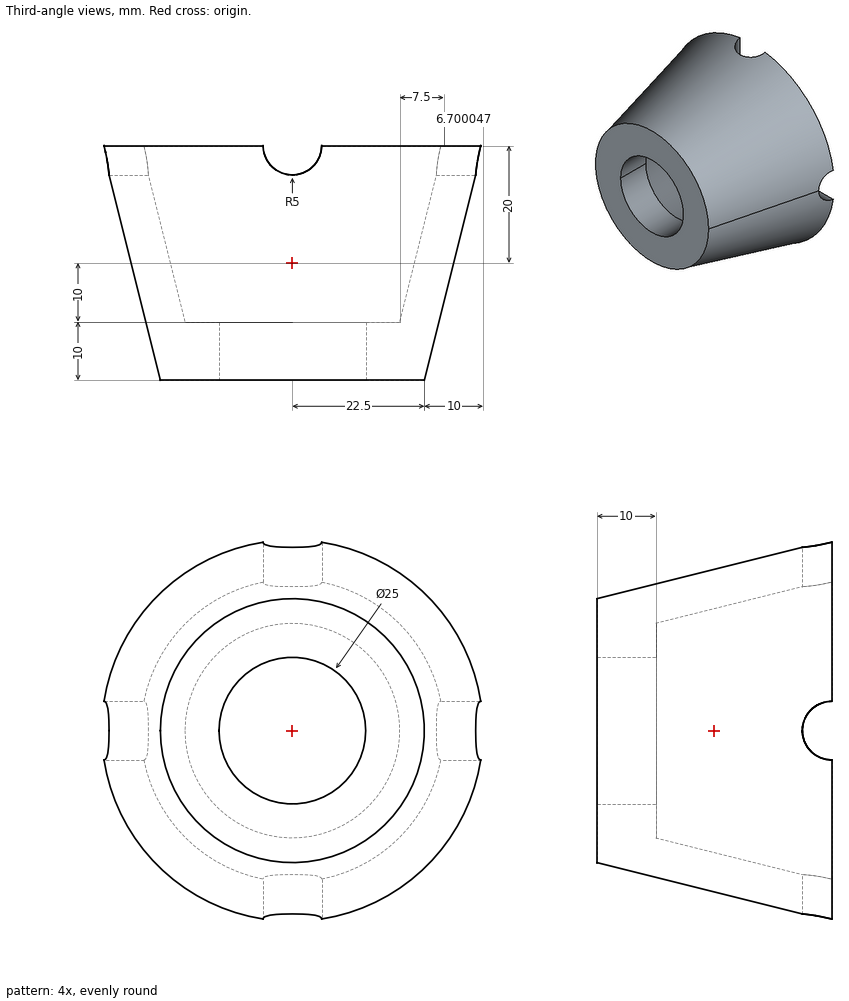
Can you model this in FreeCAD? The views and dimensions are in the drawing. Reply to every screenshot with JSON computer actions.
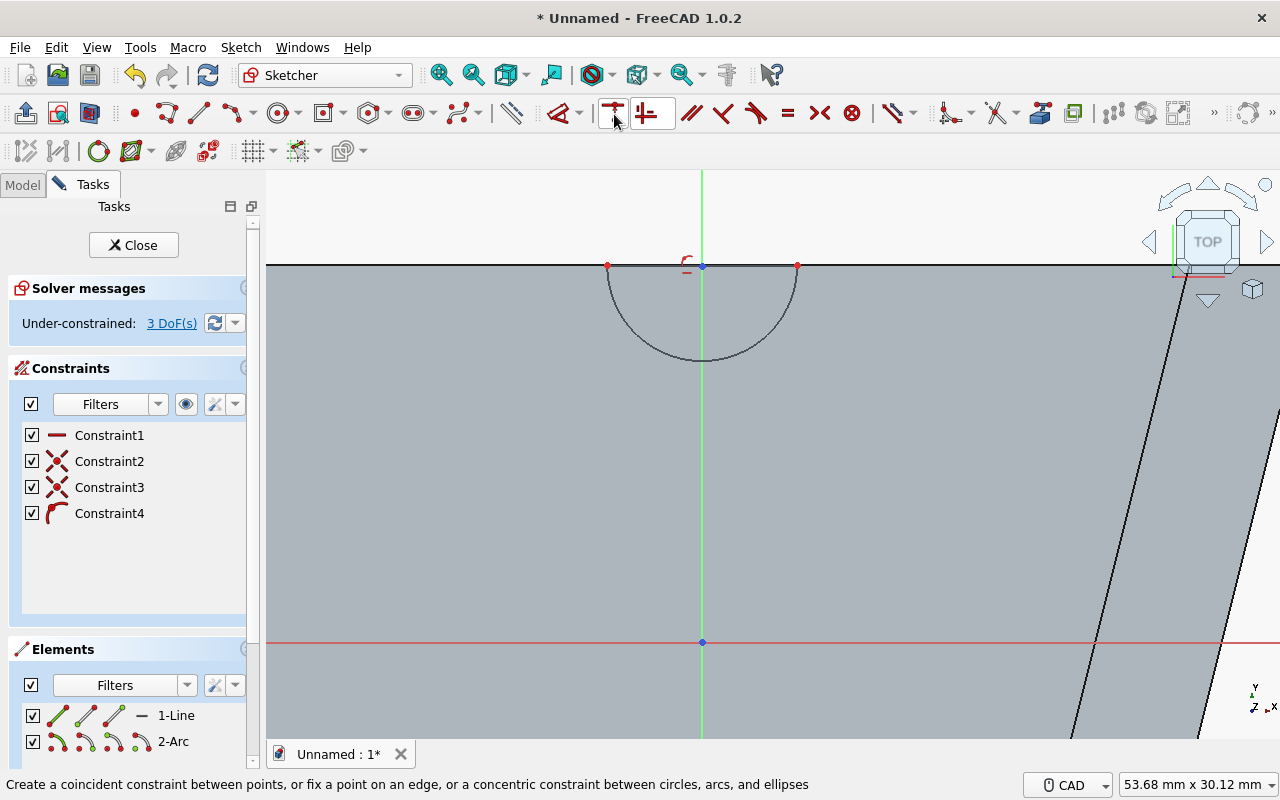
{"action": "left_click", "coordinate": [558, 114]}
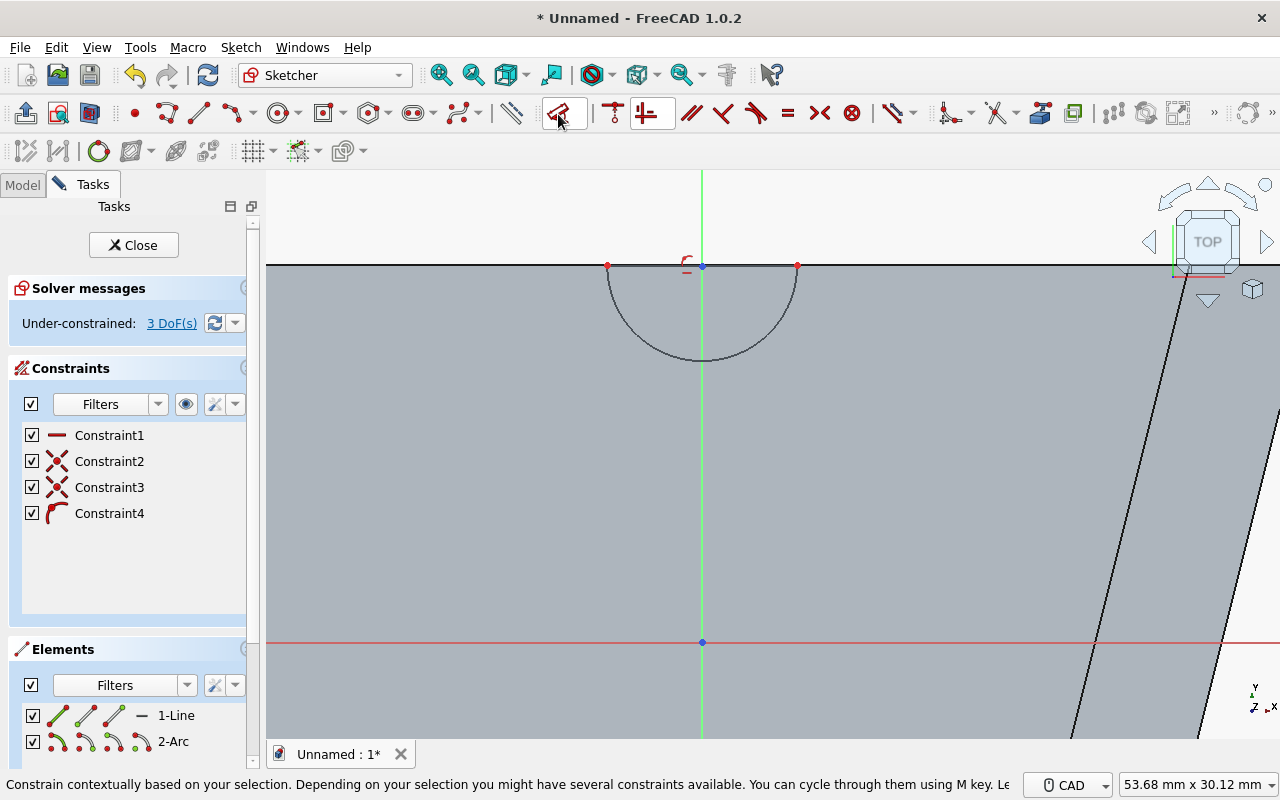
{"action": "left_click", "coordinate": [646, 343]}
{"action": "left_click", "coordinate": [627, 369]}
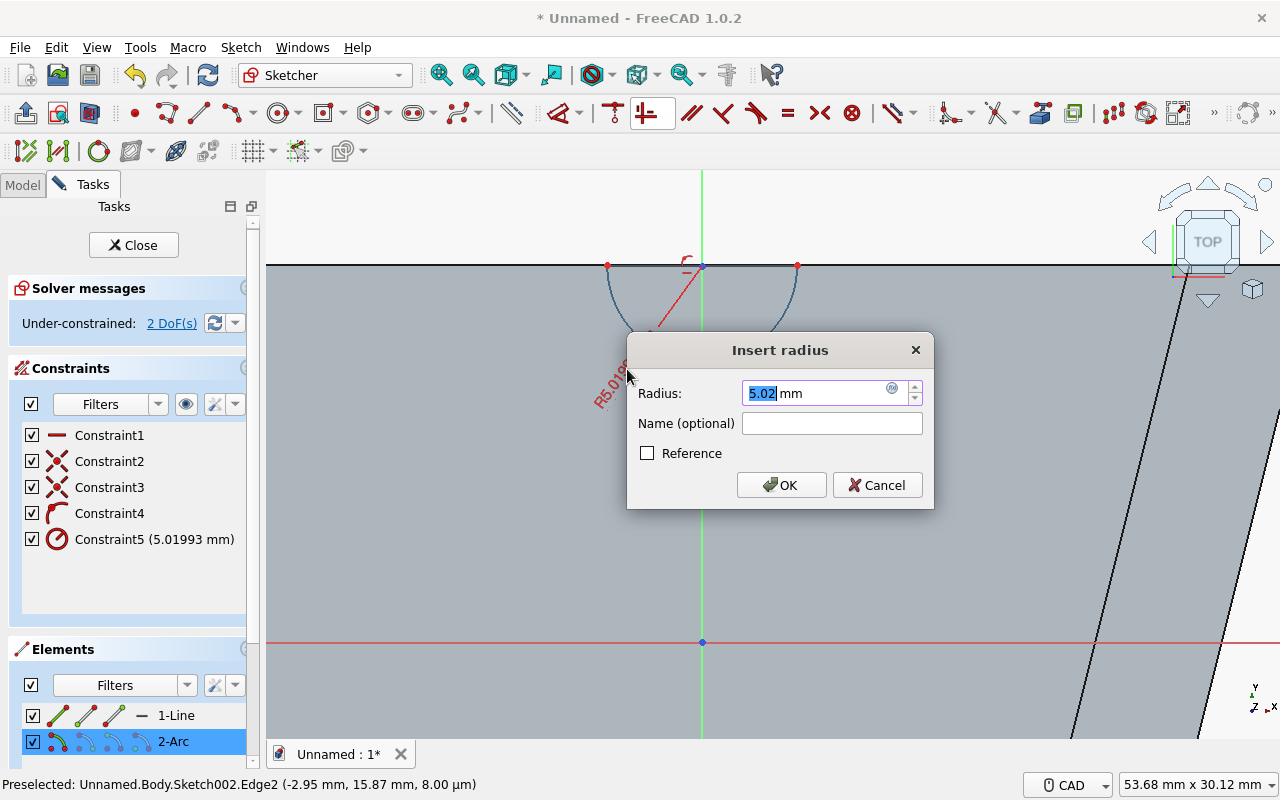
{"action": "type", "text": "5"}
{"action": "key", "text": "Return"}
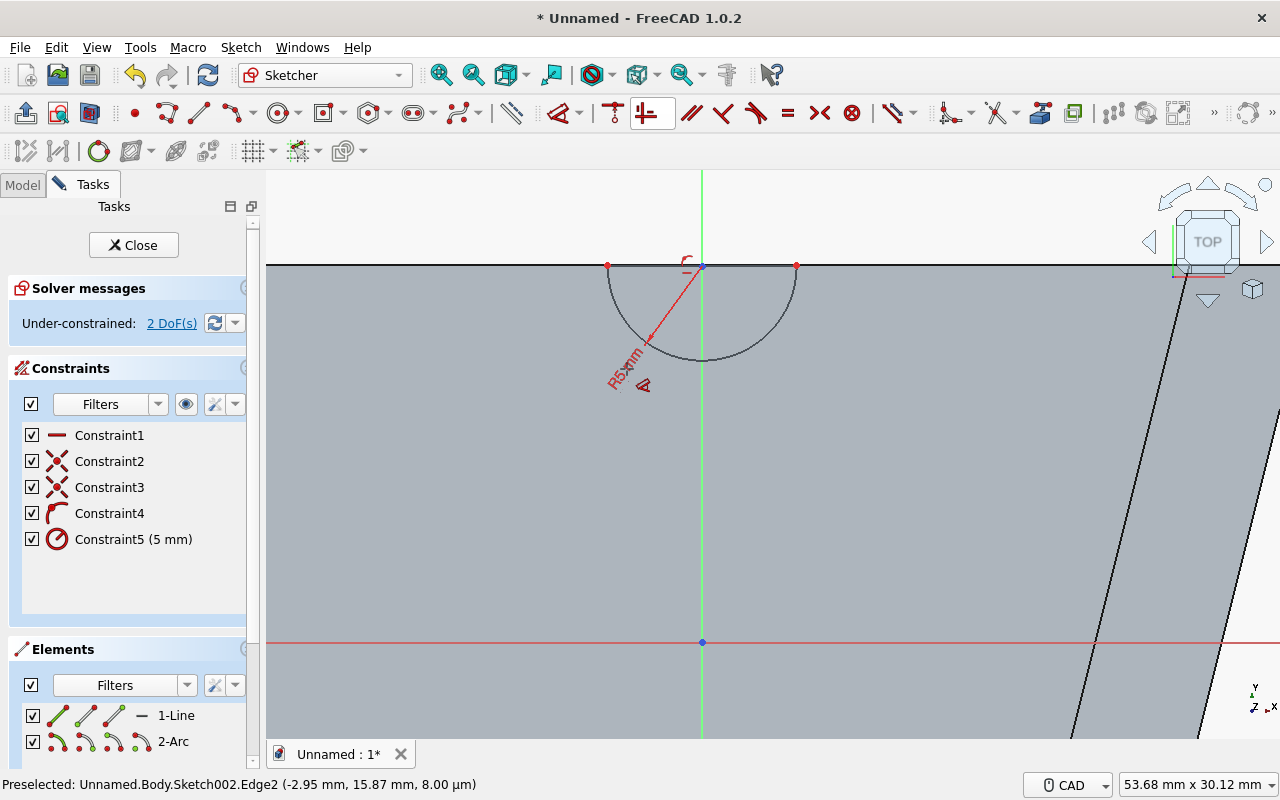
{"action": "left_click", "coordinate": [797, 266]}
{"action": "left_click", "coordinate": [831, 454]}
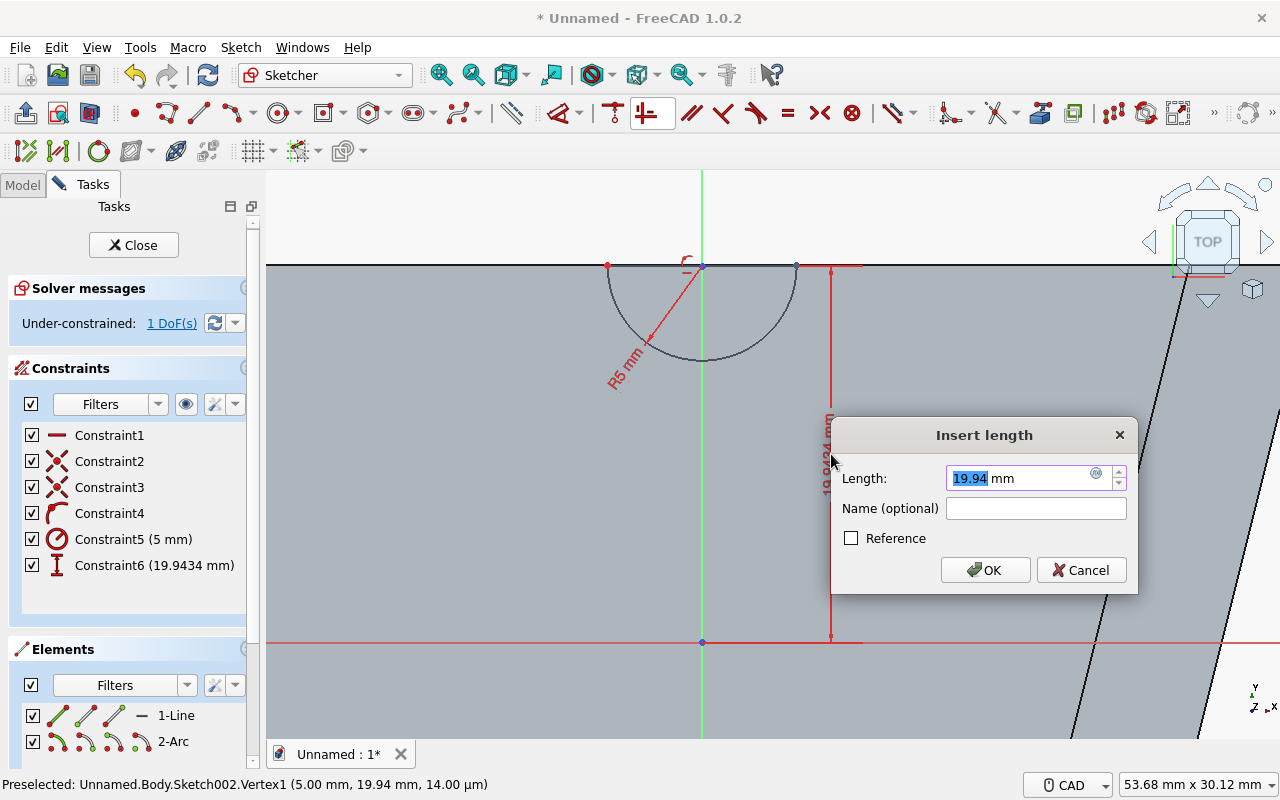
{"action": "type", "text": "20"}
{"action": "key", "text": "Return"}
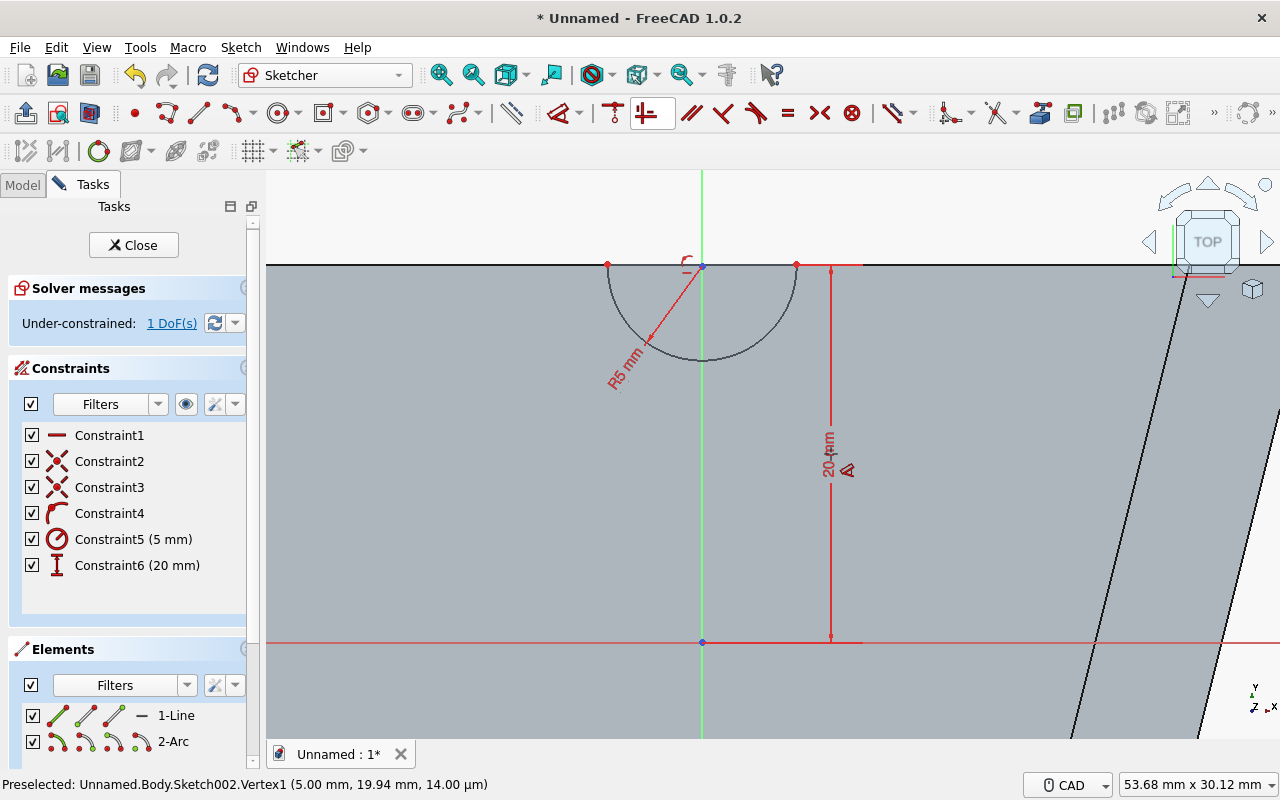
{"action": "left_click", "coordinate": [702, 266]}
{"action": "left_click", "coordinate": [736, 454]}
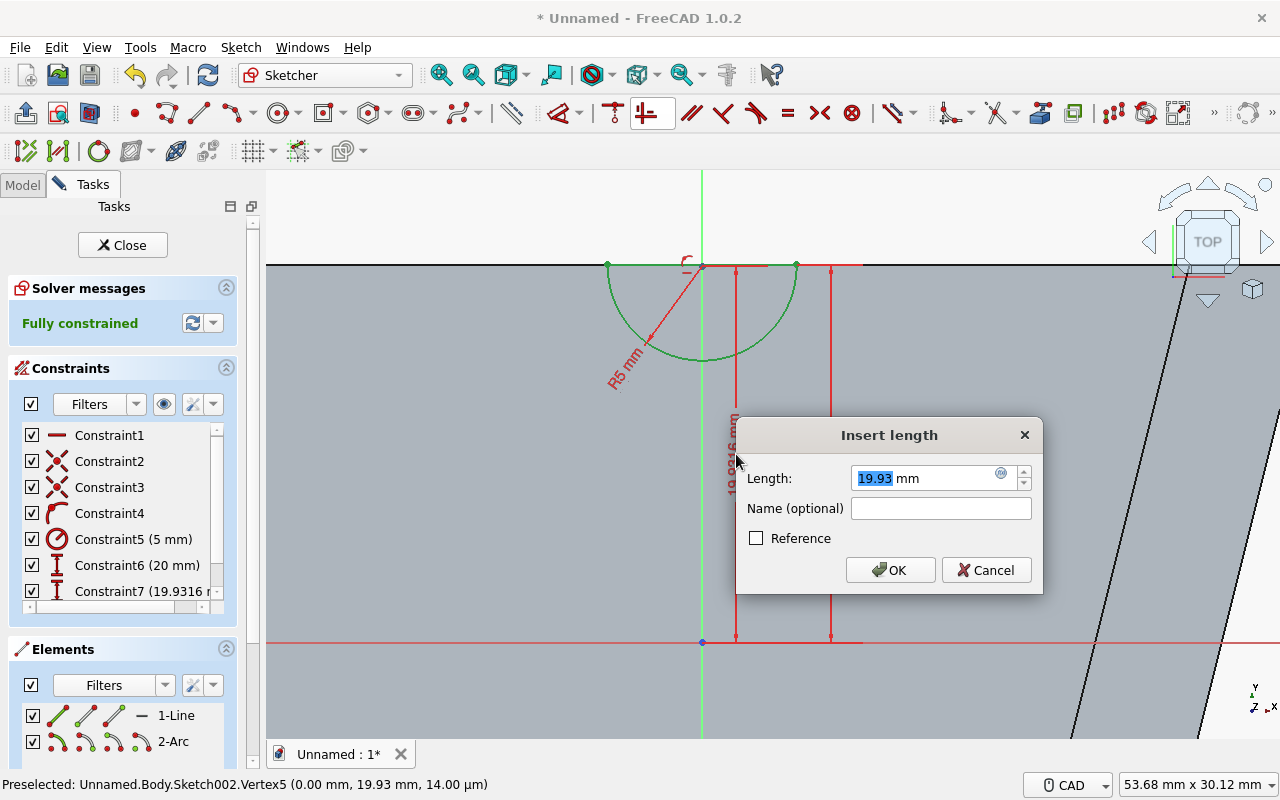
{"action": "type", "text": "20"}
{"action": "key", "text": "Return"}
{"action": "key", "text": "Escape"}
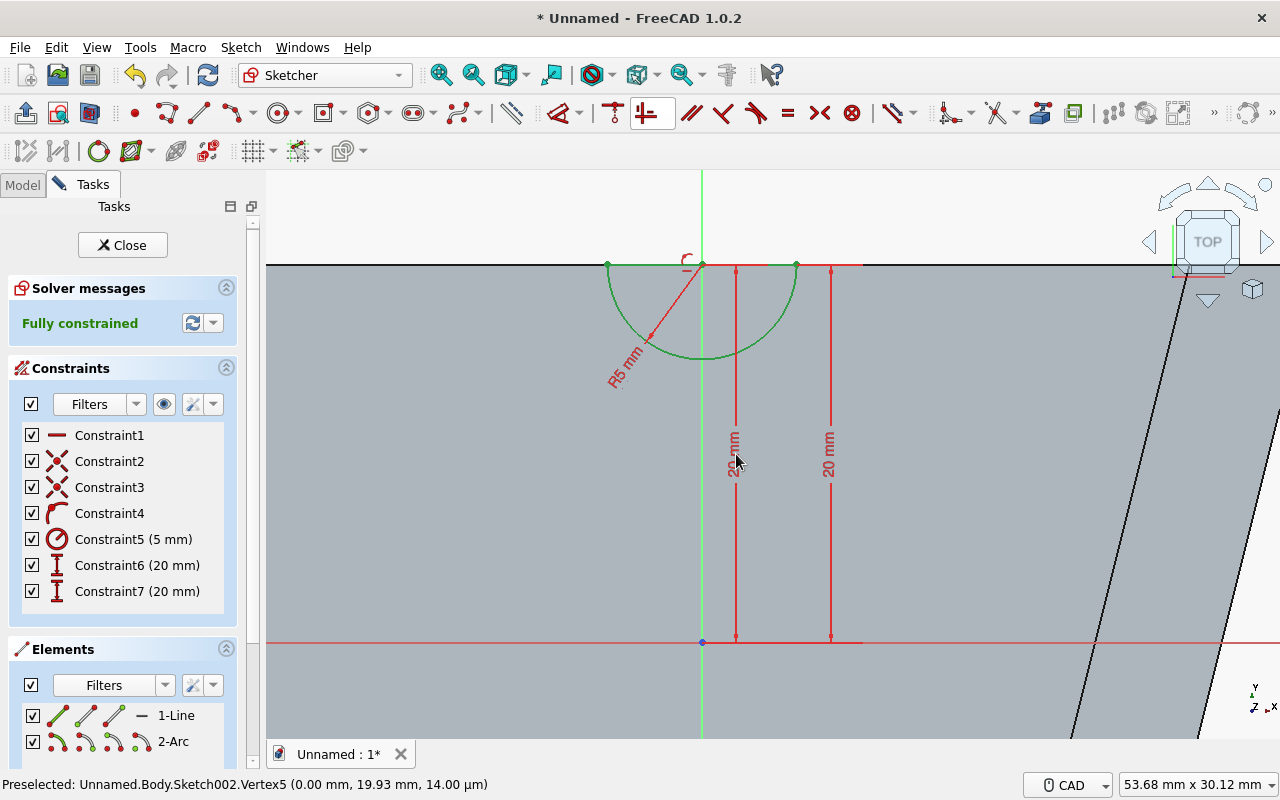
{"action": "left_click", "coordinate": [123, 245]}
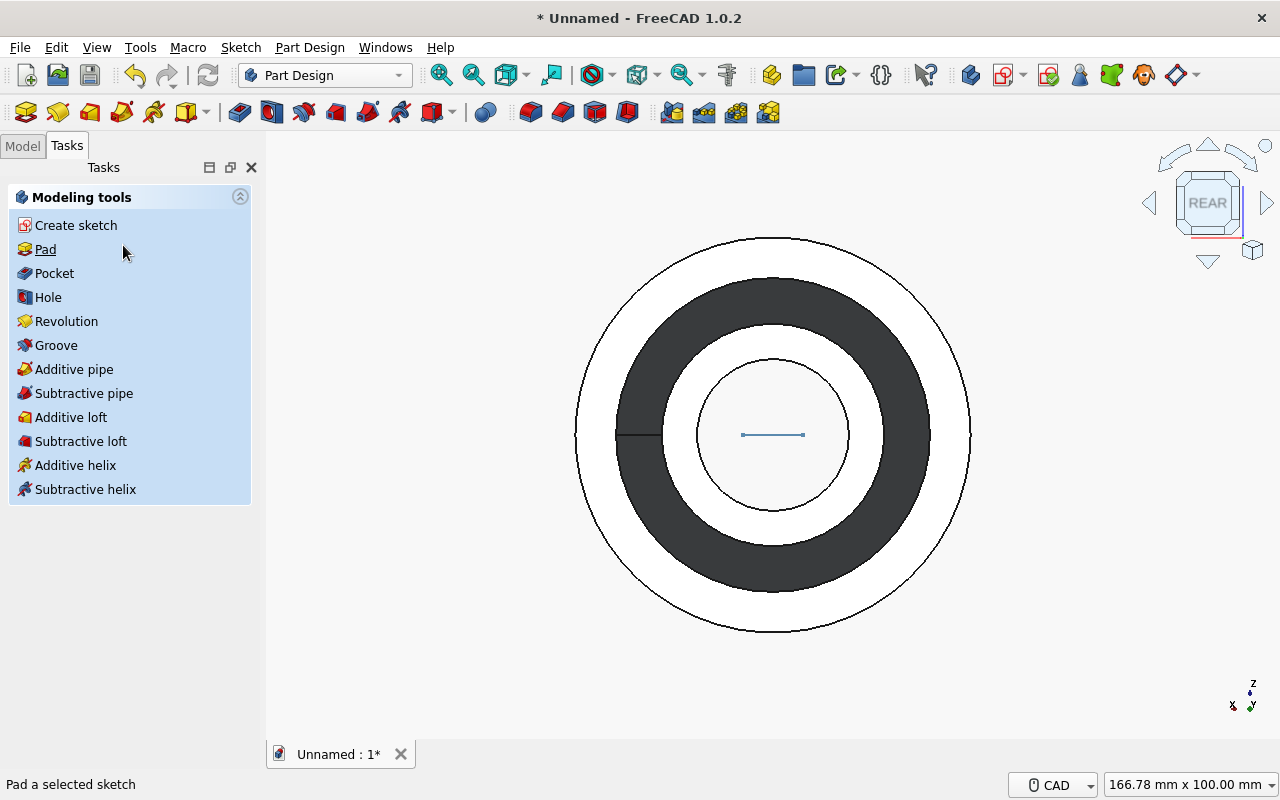
{"action": "left_click", "coordinate": [240, 112]}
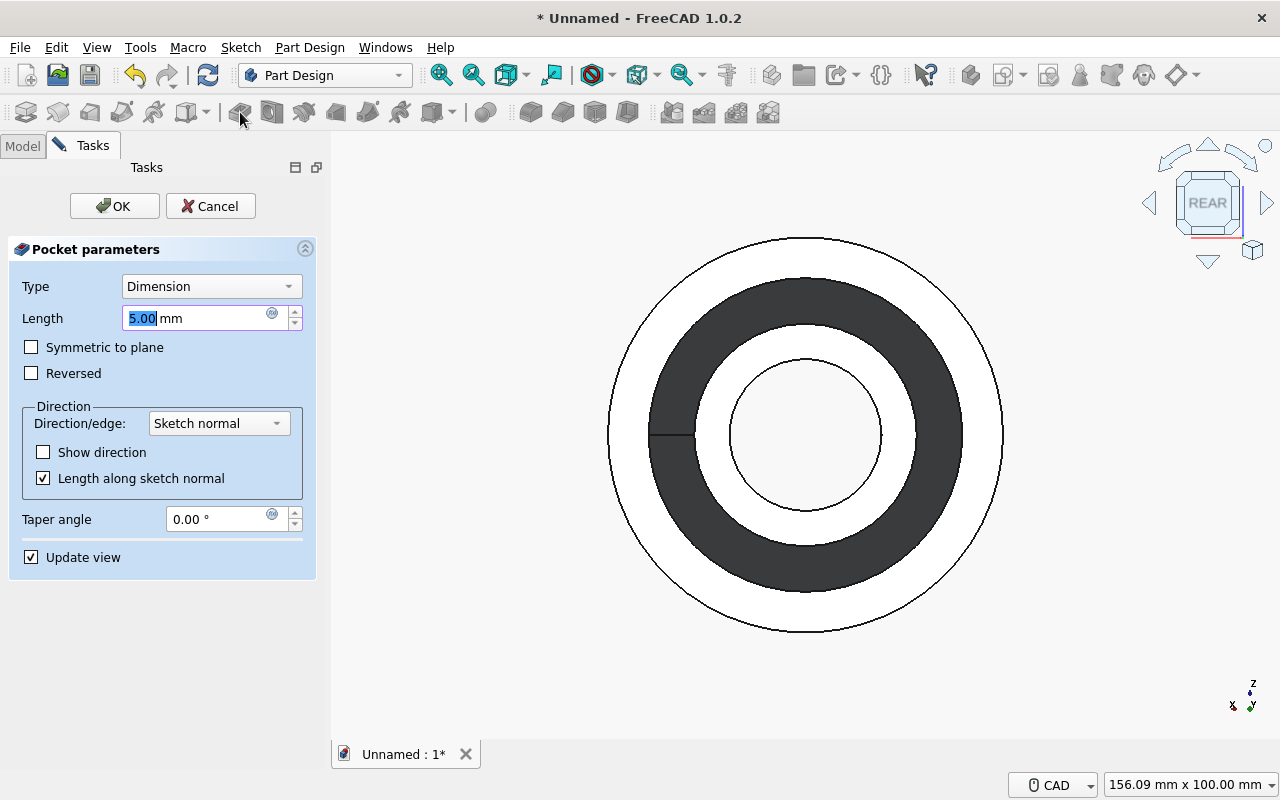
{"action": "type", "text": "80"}
{"action": "key", "text": "Tab"}